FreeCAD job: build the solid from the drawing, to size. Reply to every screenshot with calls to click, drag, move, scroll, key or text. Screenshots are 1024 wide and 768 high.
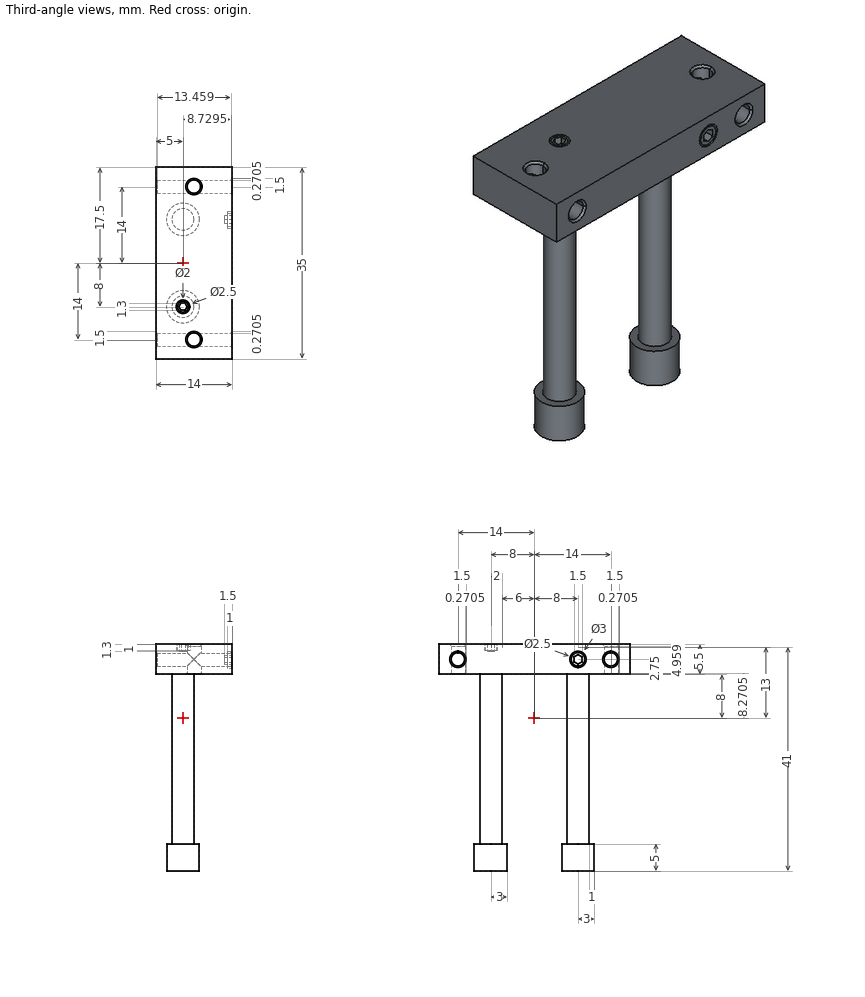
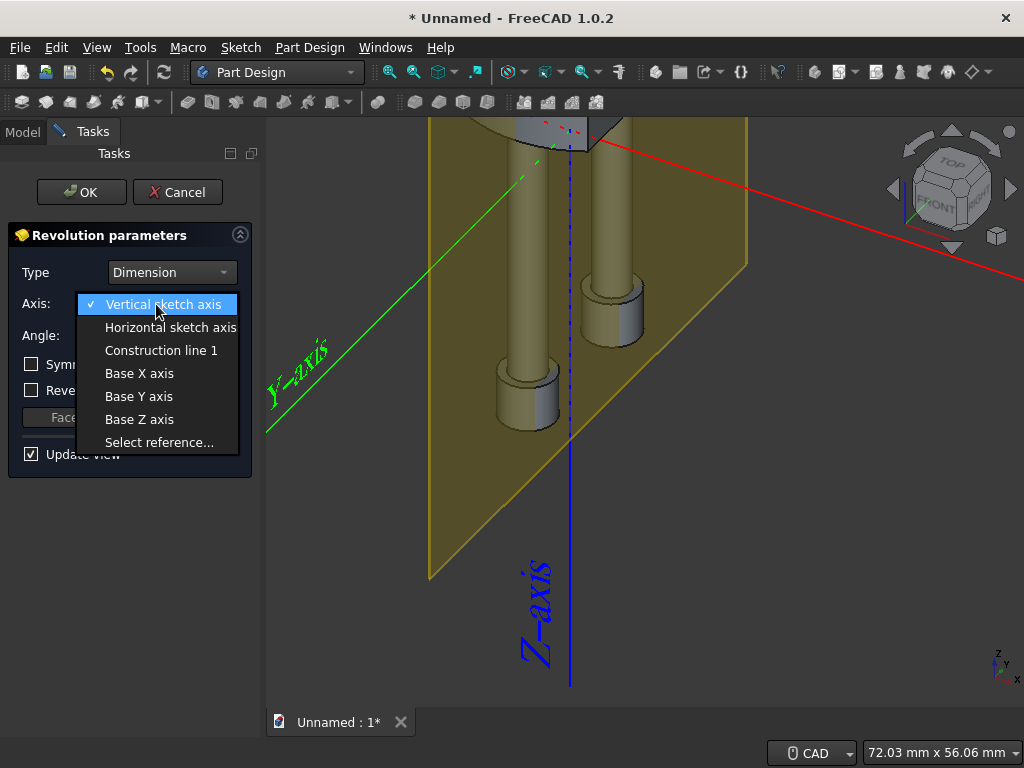
click(156, 350)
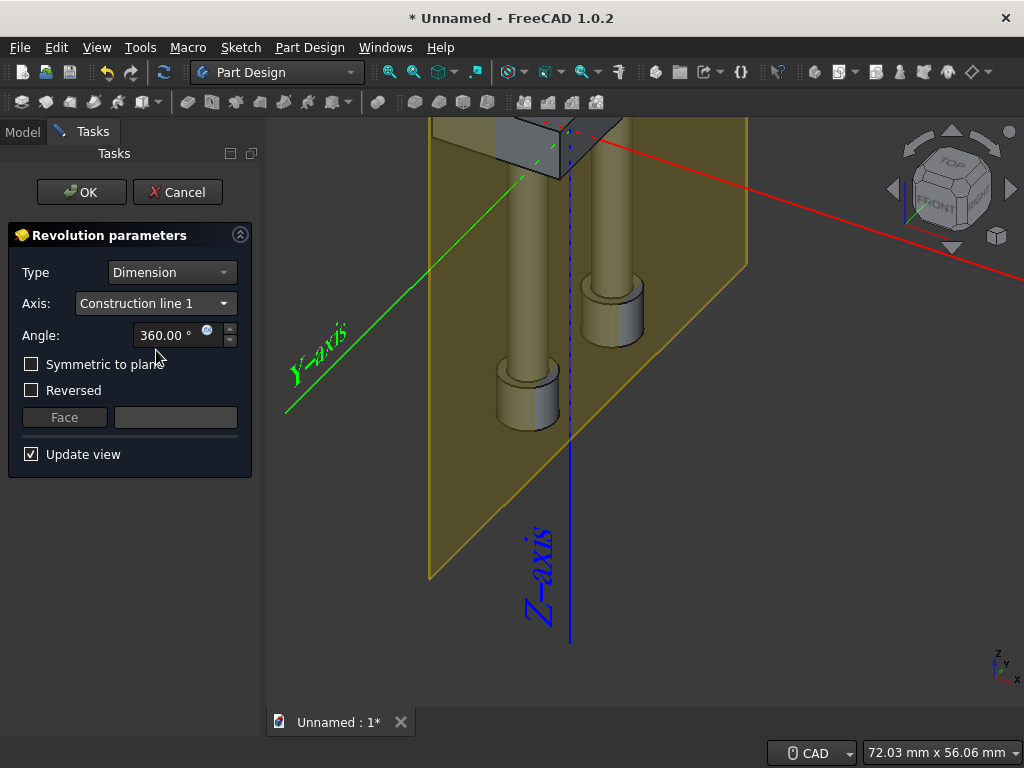
click(82, 192)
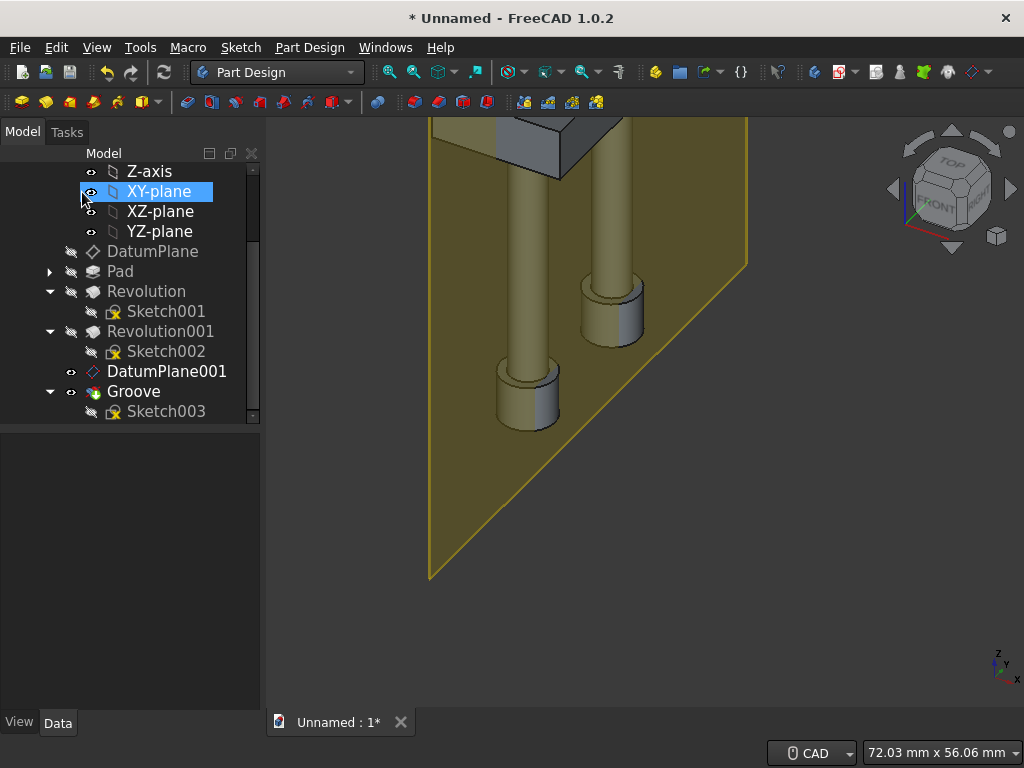
click(116, 372)
key(space)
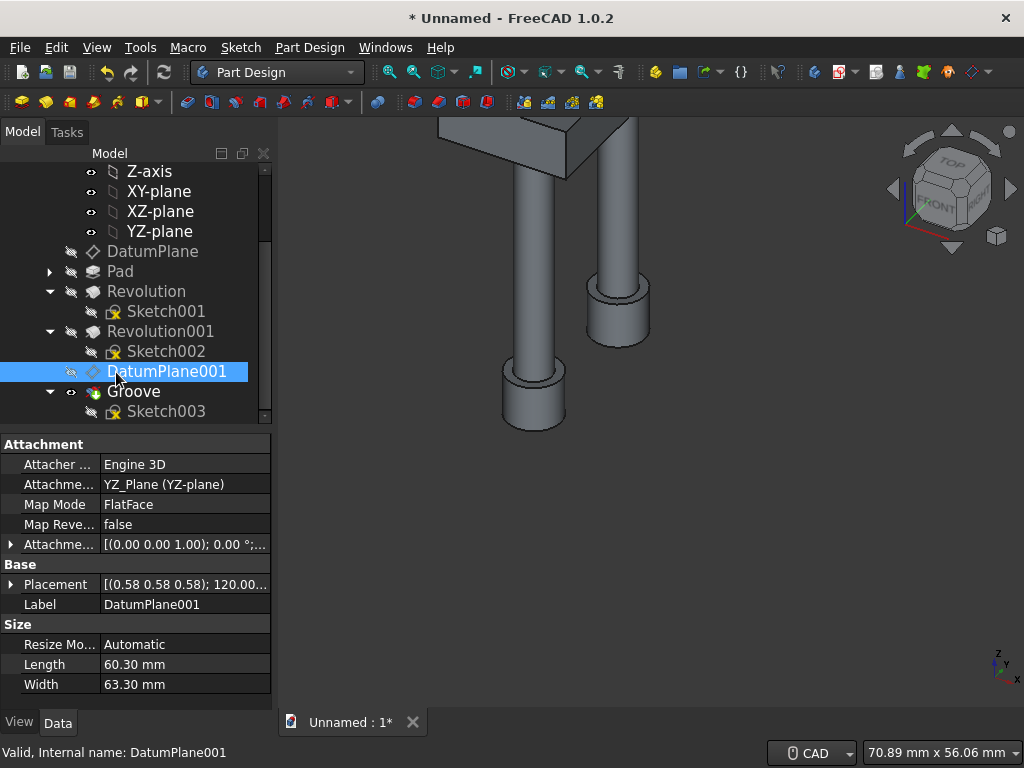
click(390, 72)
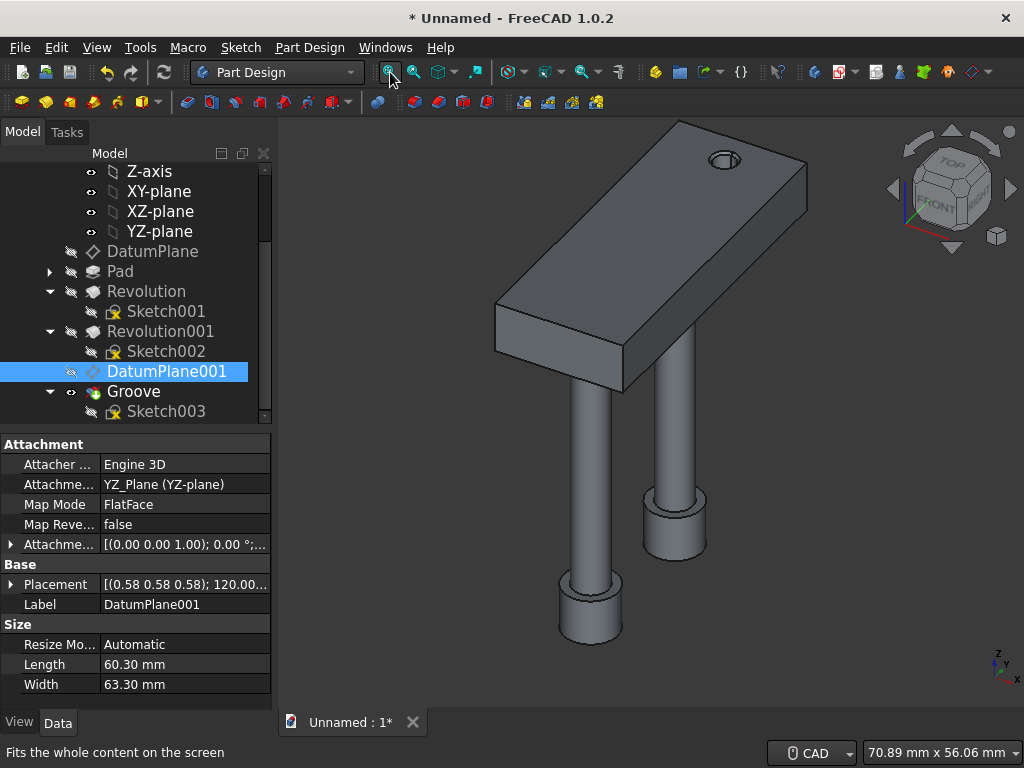
scroll(160, 287, down, 3)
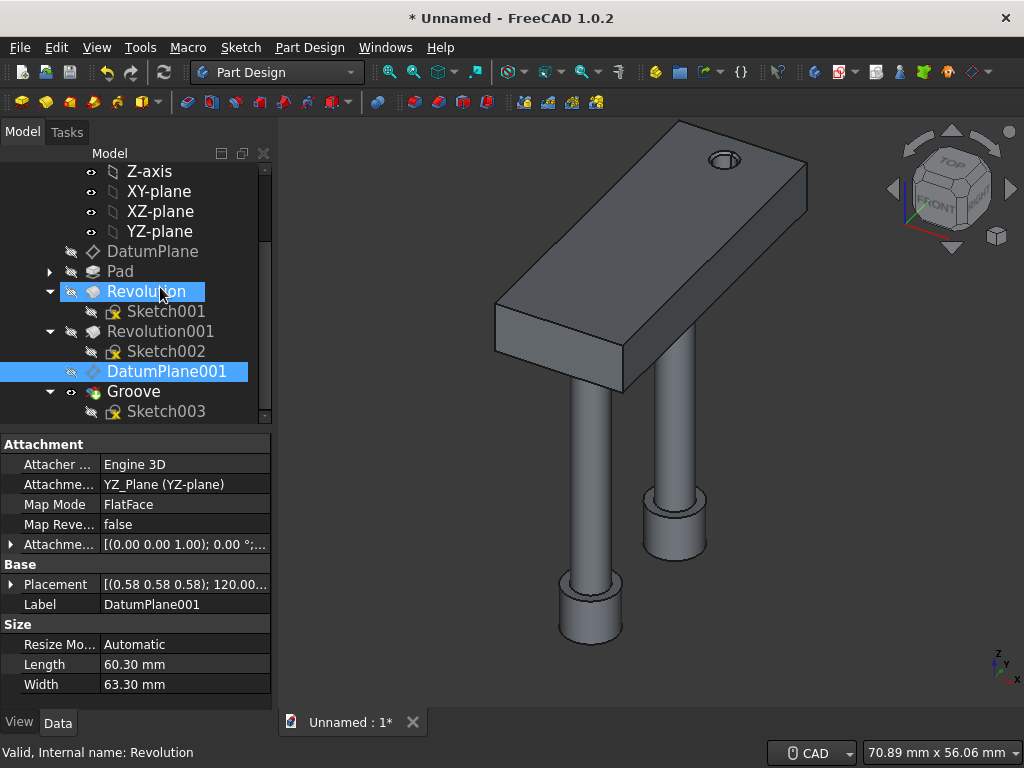
scroll(160, 287, up, 15)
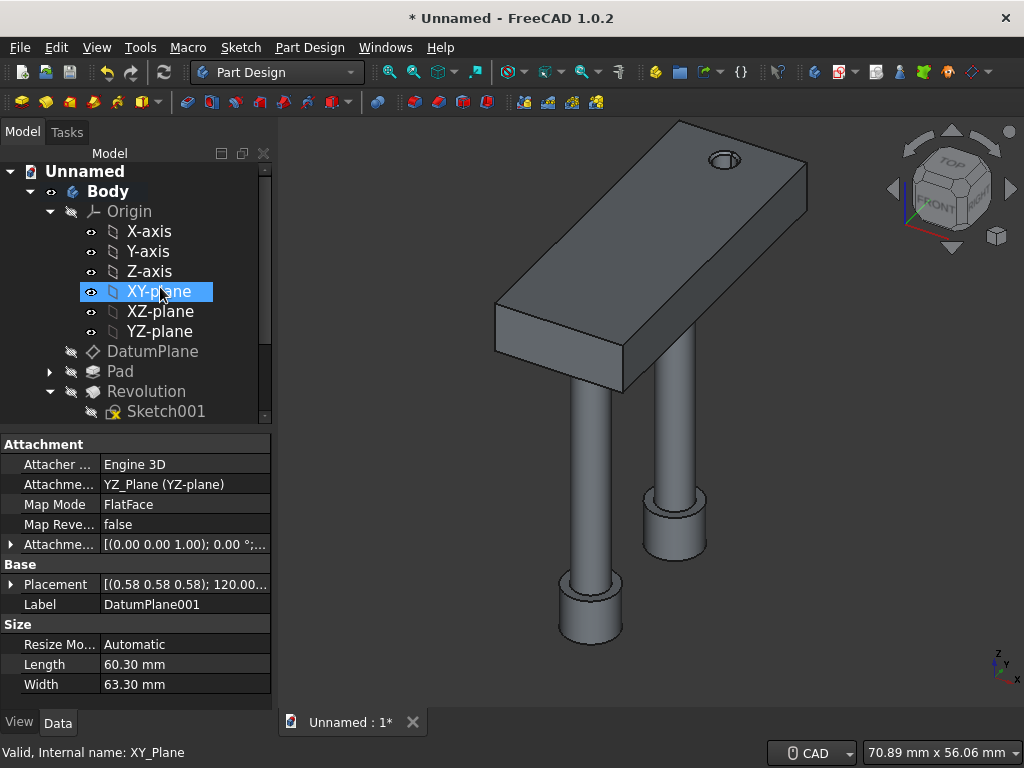
click(136, 332)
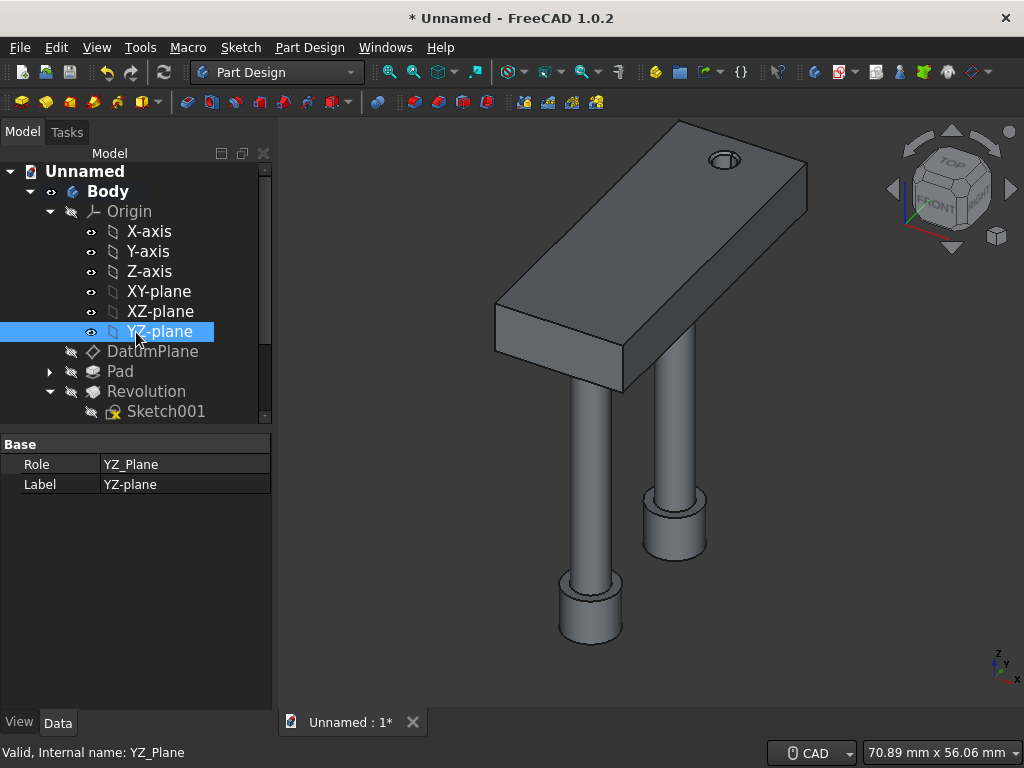
click(972, 72)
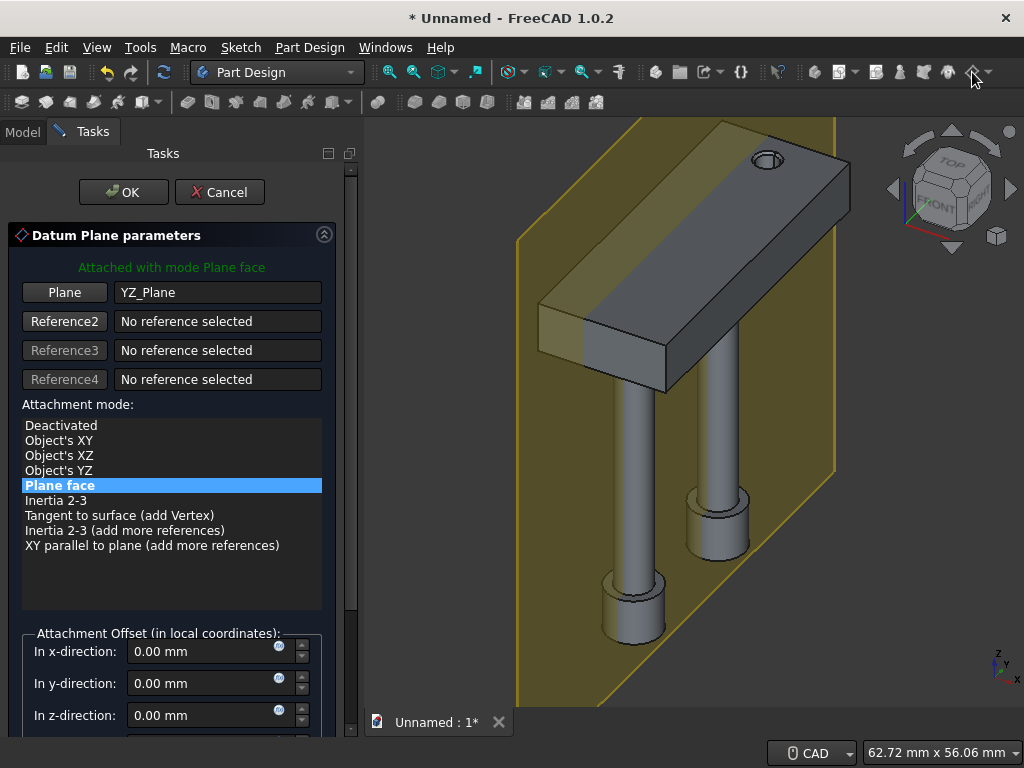
triple_click(210, 715)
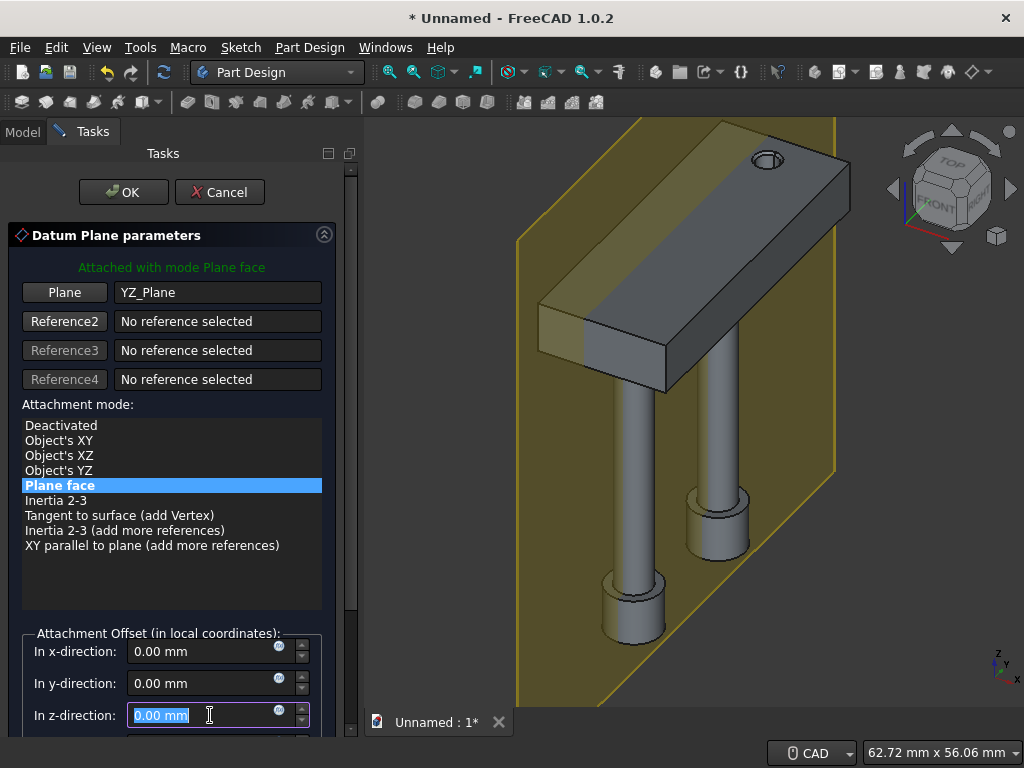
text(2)
key(Tab)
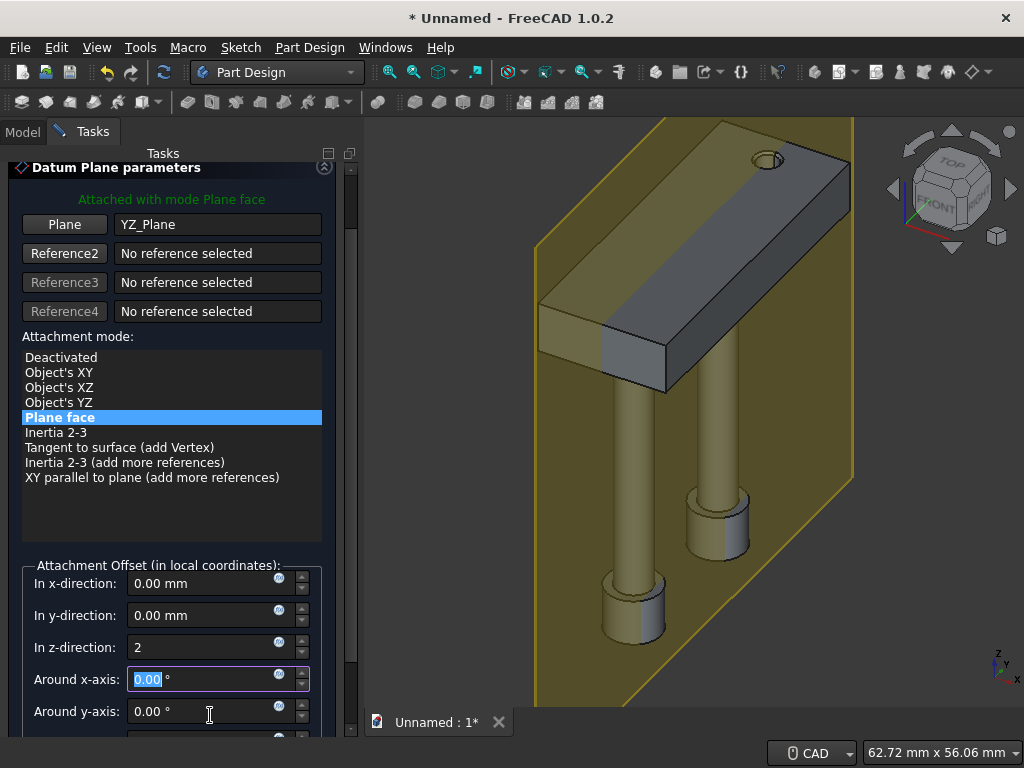
scroll(351, 450, up, 2)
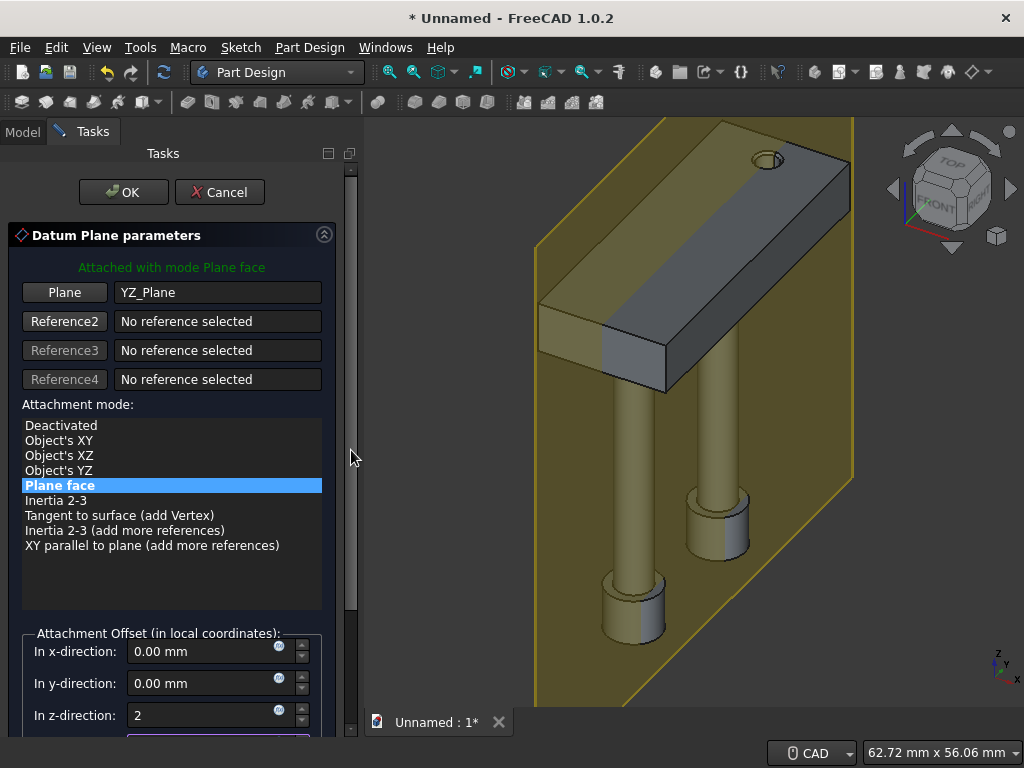
click(124, 192)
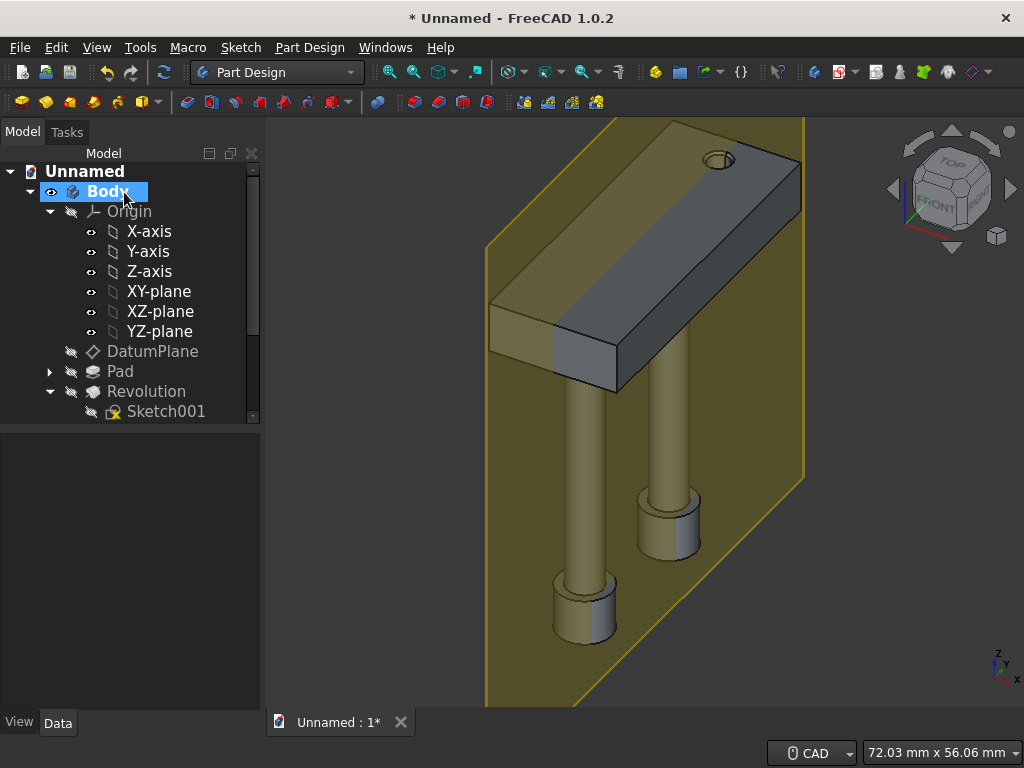
scroll(100, 287, down, 3)